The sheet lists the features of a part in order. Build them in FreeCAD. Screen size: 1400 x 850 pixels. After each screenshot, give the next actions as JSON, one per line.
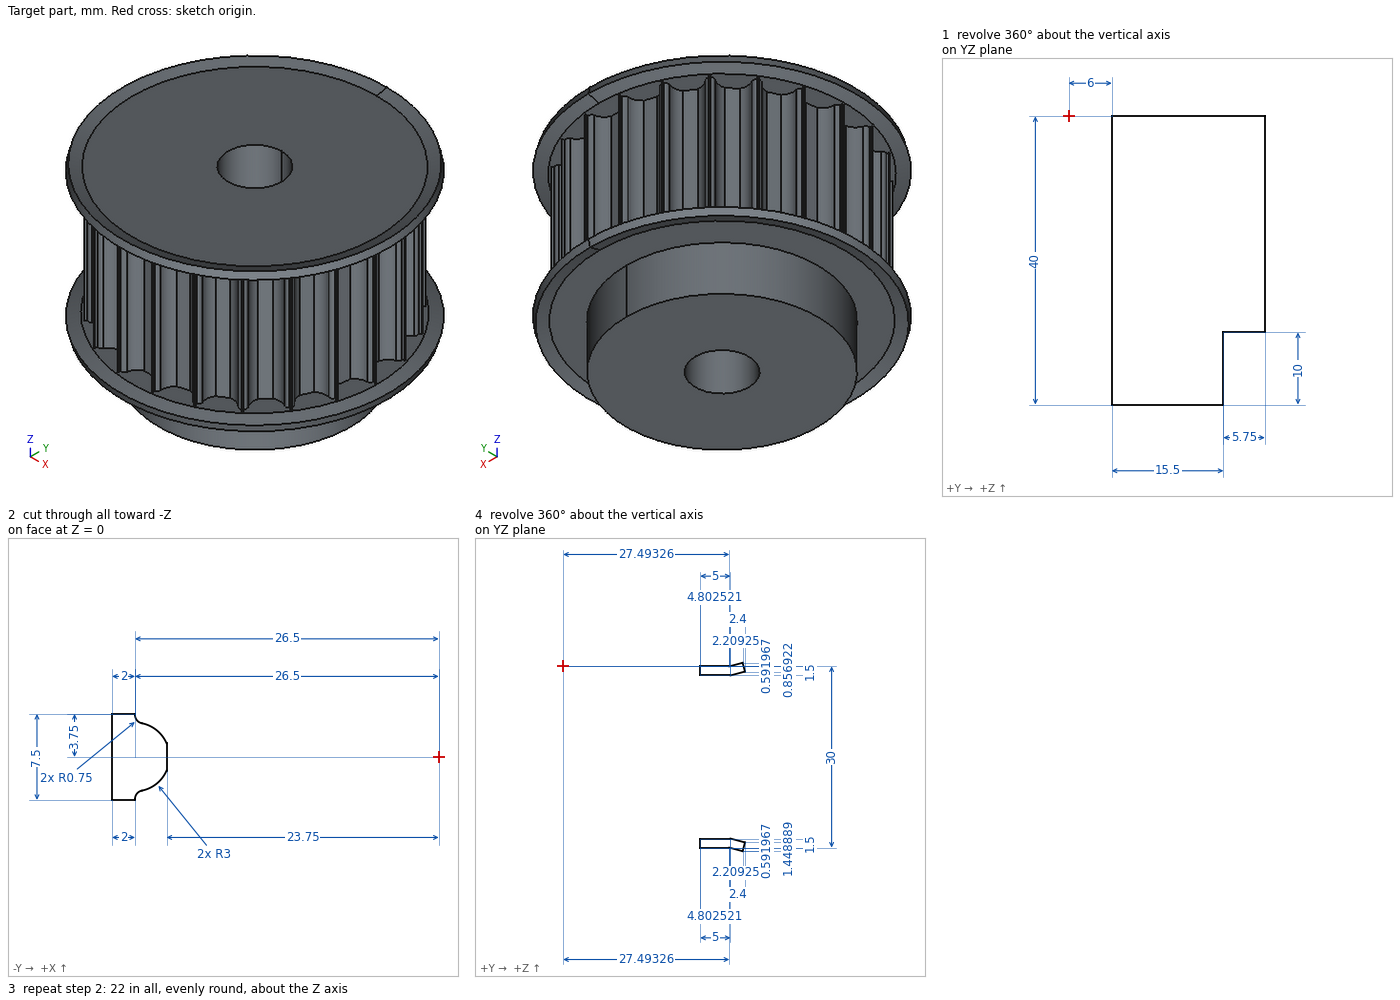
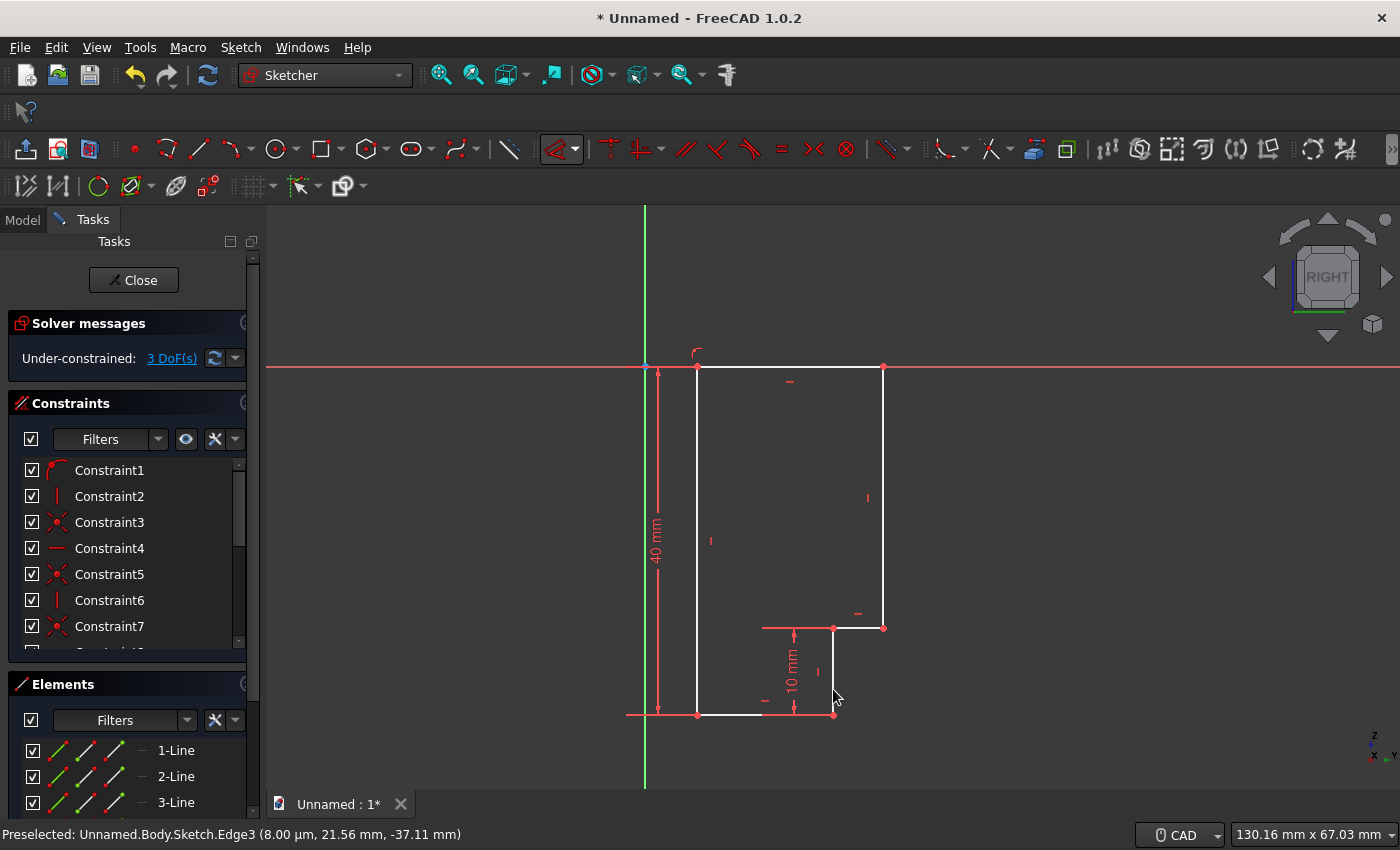
{"action": "left_click", "coordinate": [697, 367]}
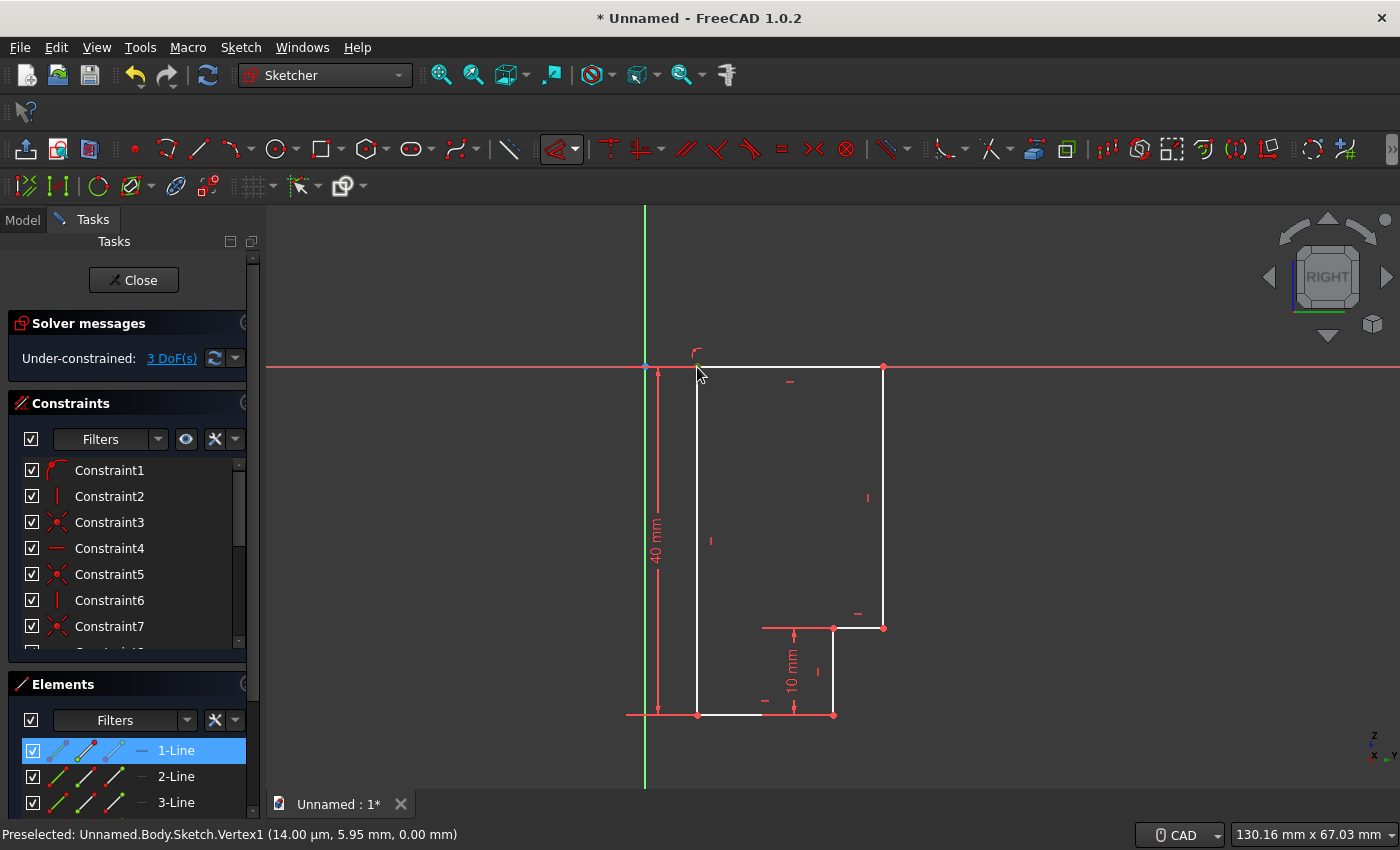
{"action": "left_click", "coordinate": [578, 150]}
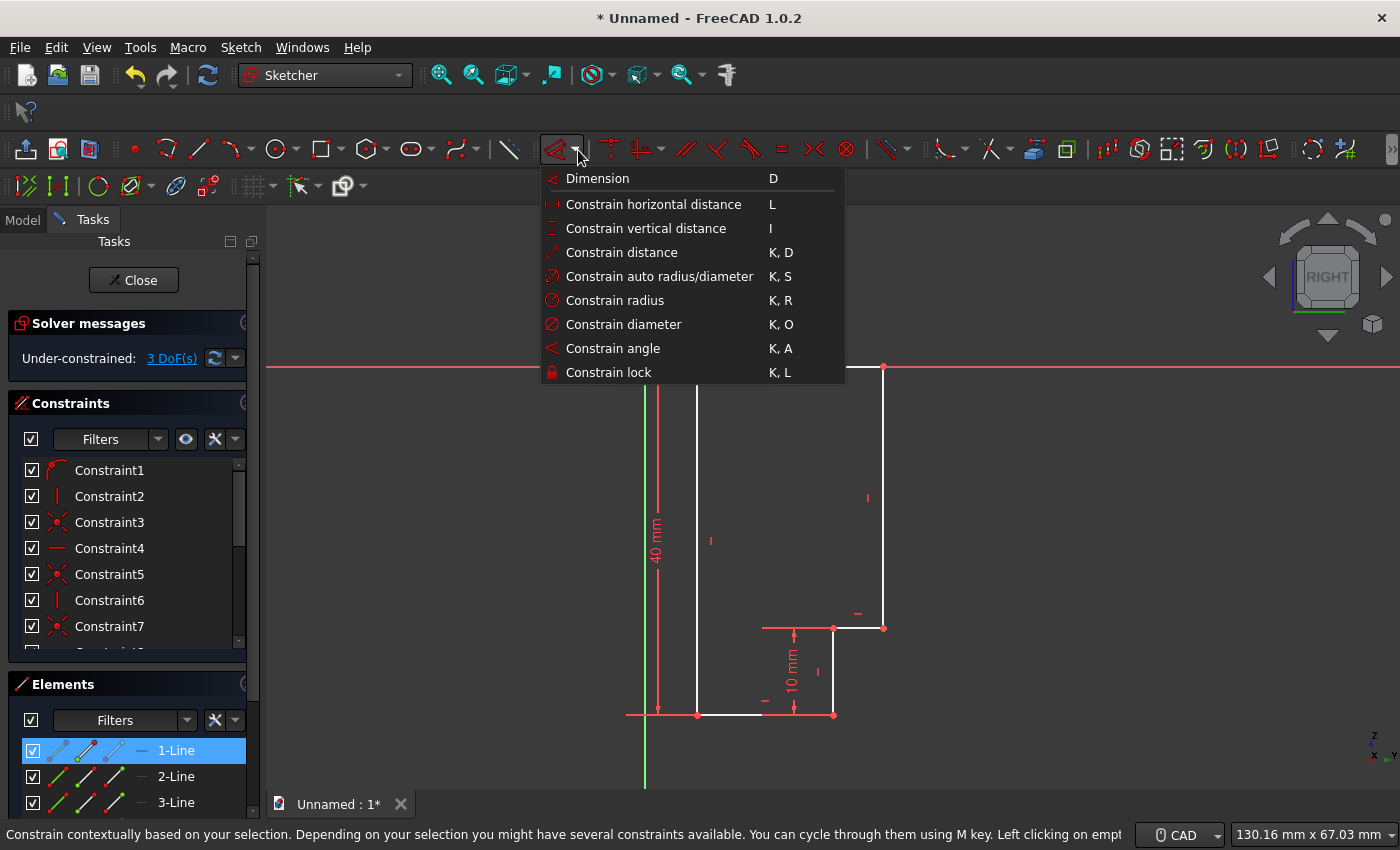
{"action": "left_click", "coordinate": [693, 204]}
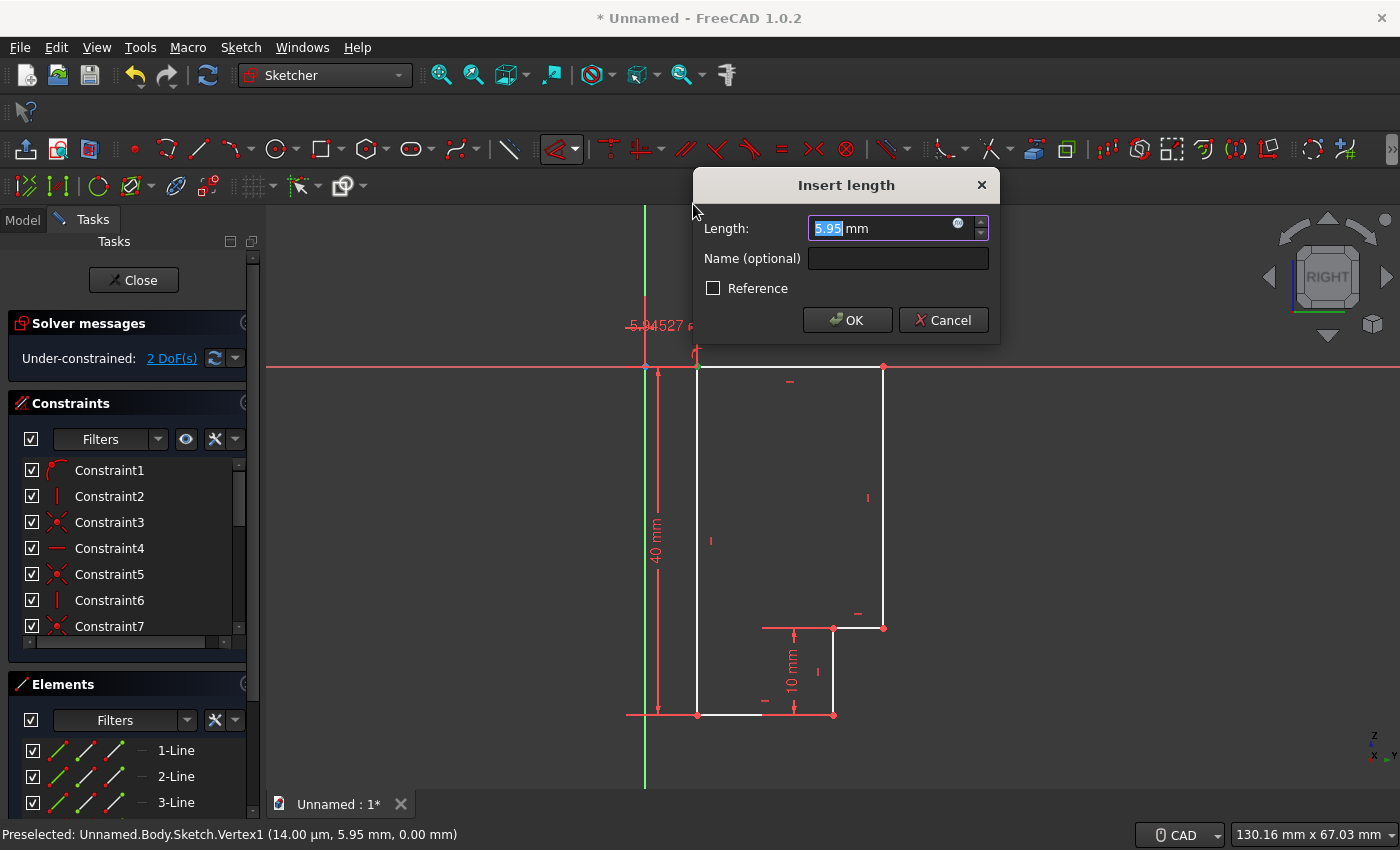
{"action": "type", "text": "6"}
{"action": "key", "text": "Return"}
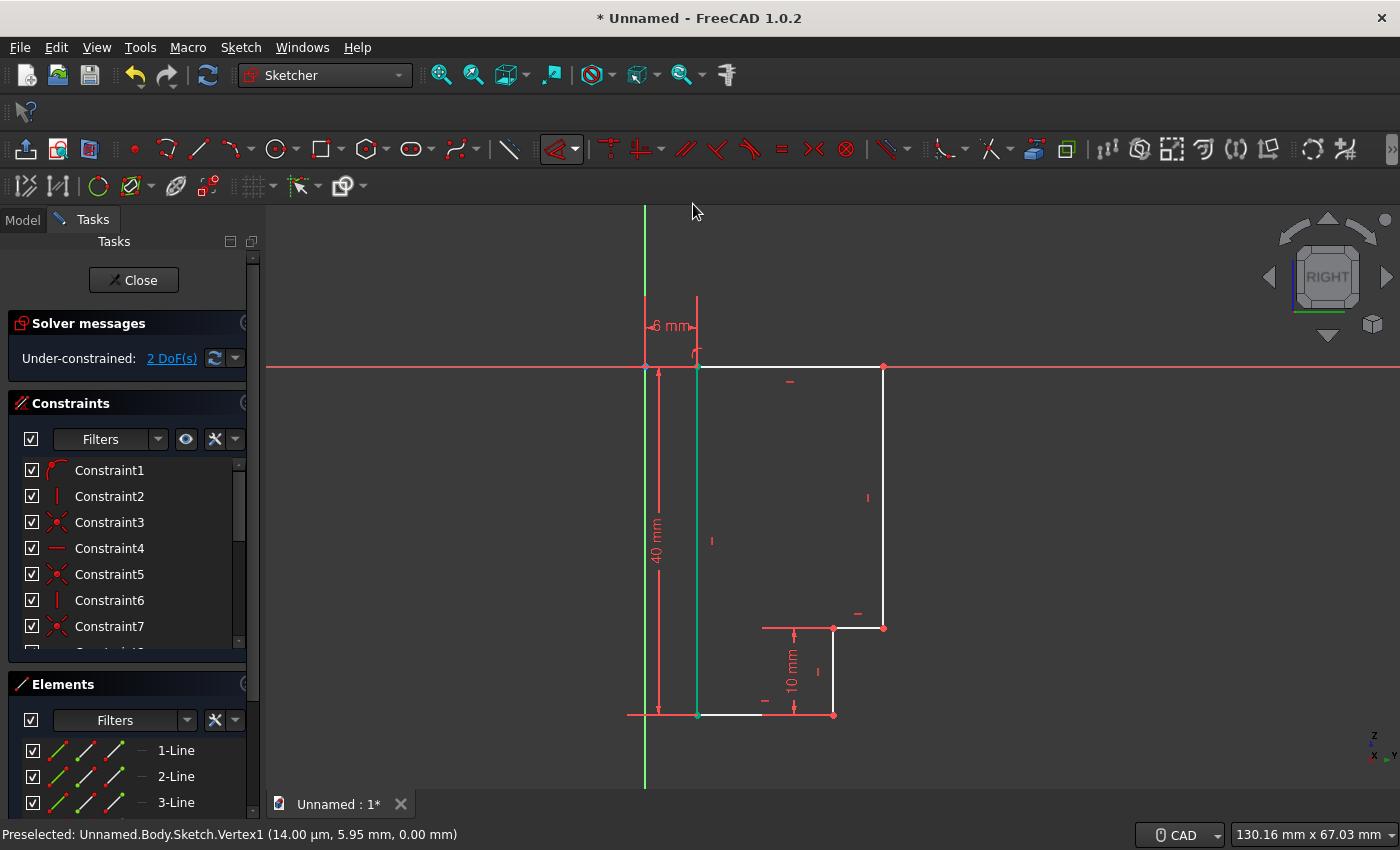
{"action": "left_click", "coordinate": [738, 715]}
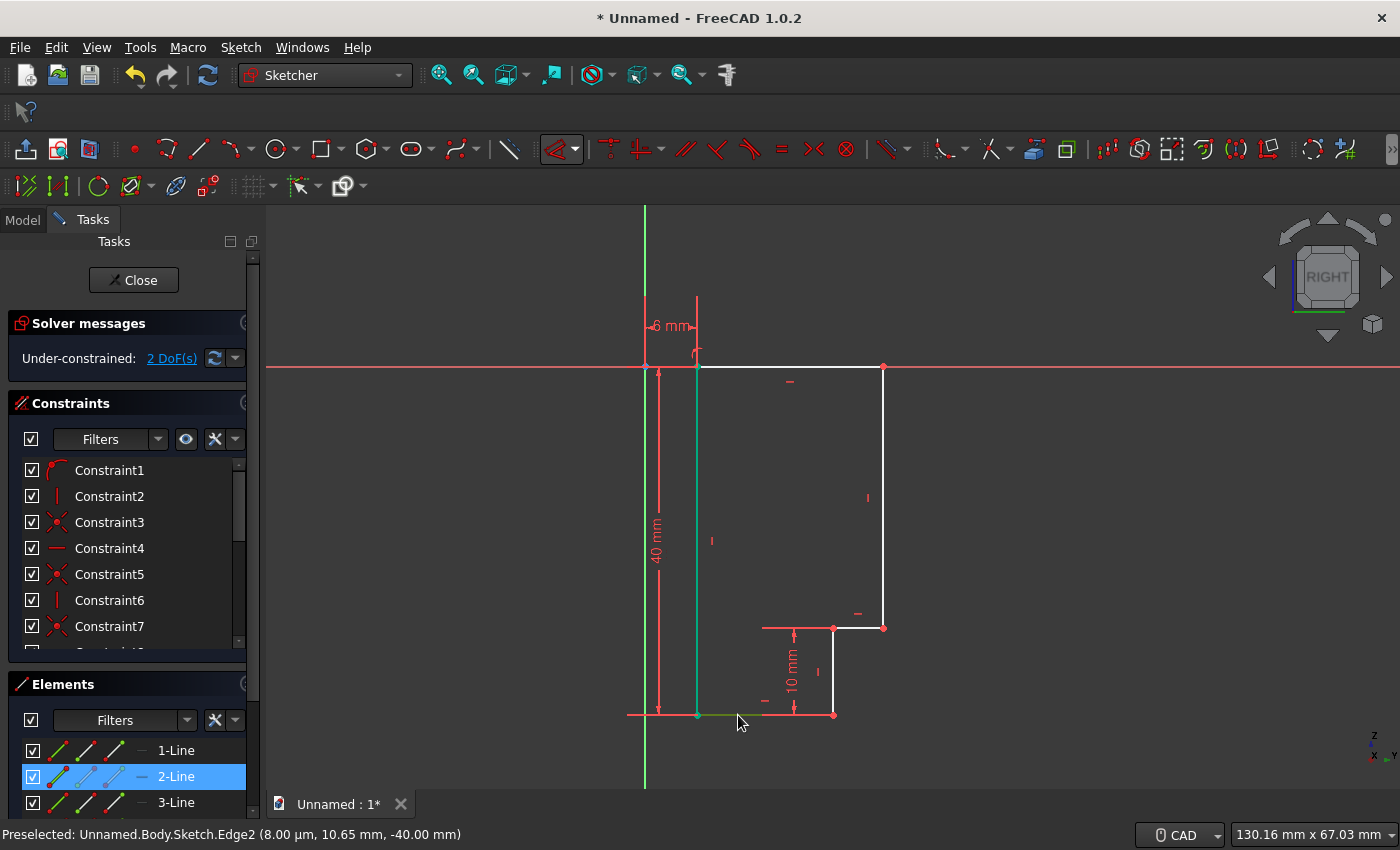
{"action": "left_click", "coordinate": [578, 150]}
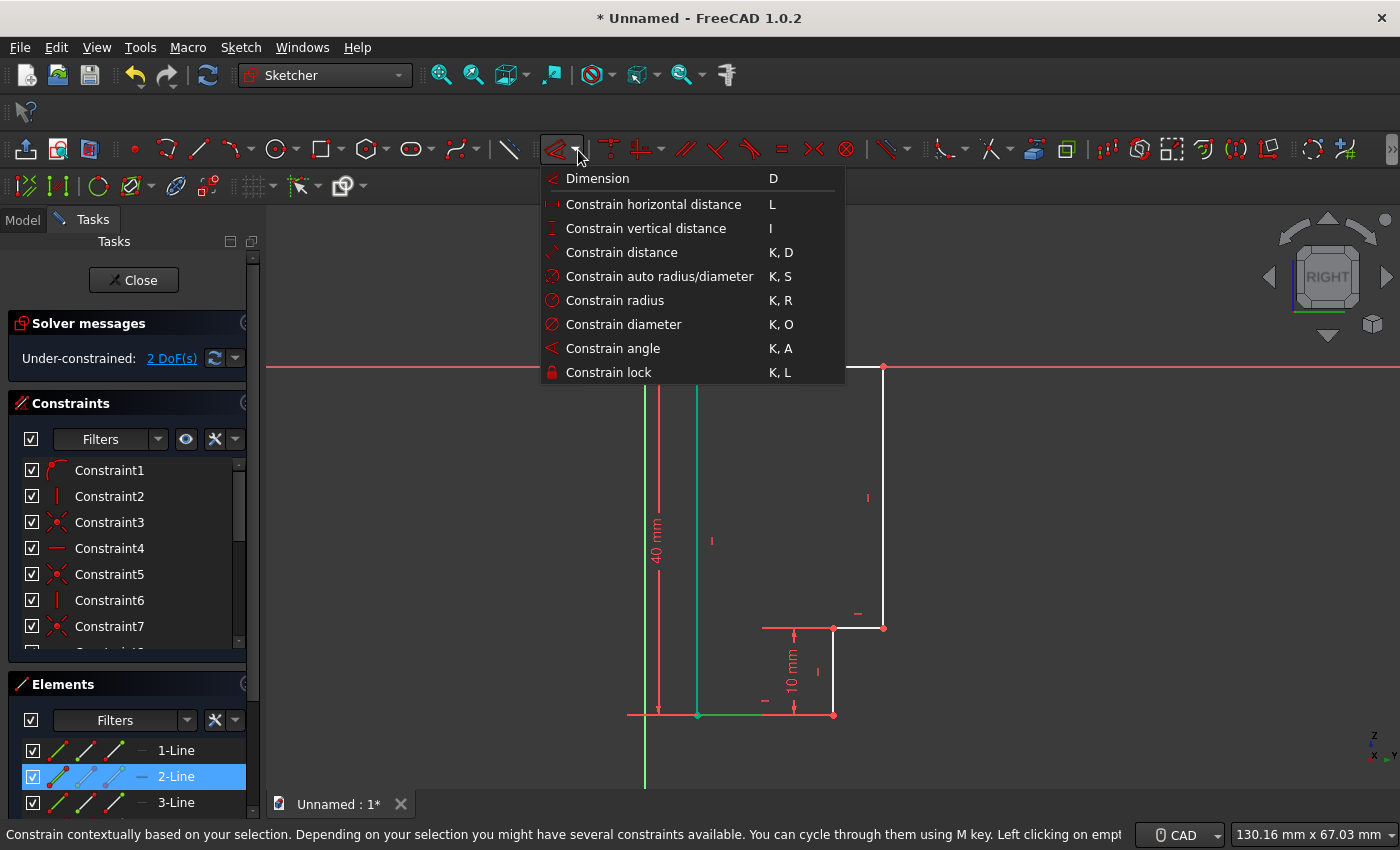
{"action": "left_click", "coordinate": [693, 204]}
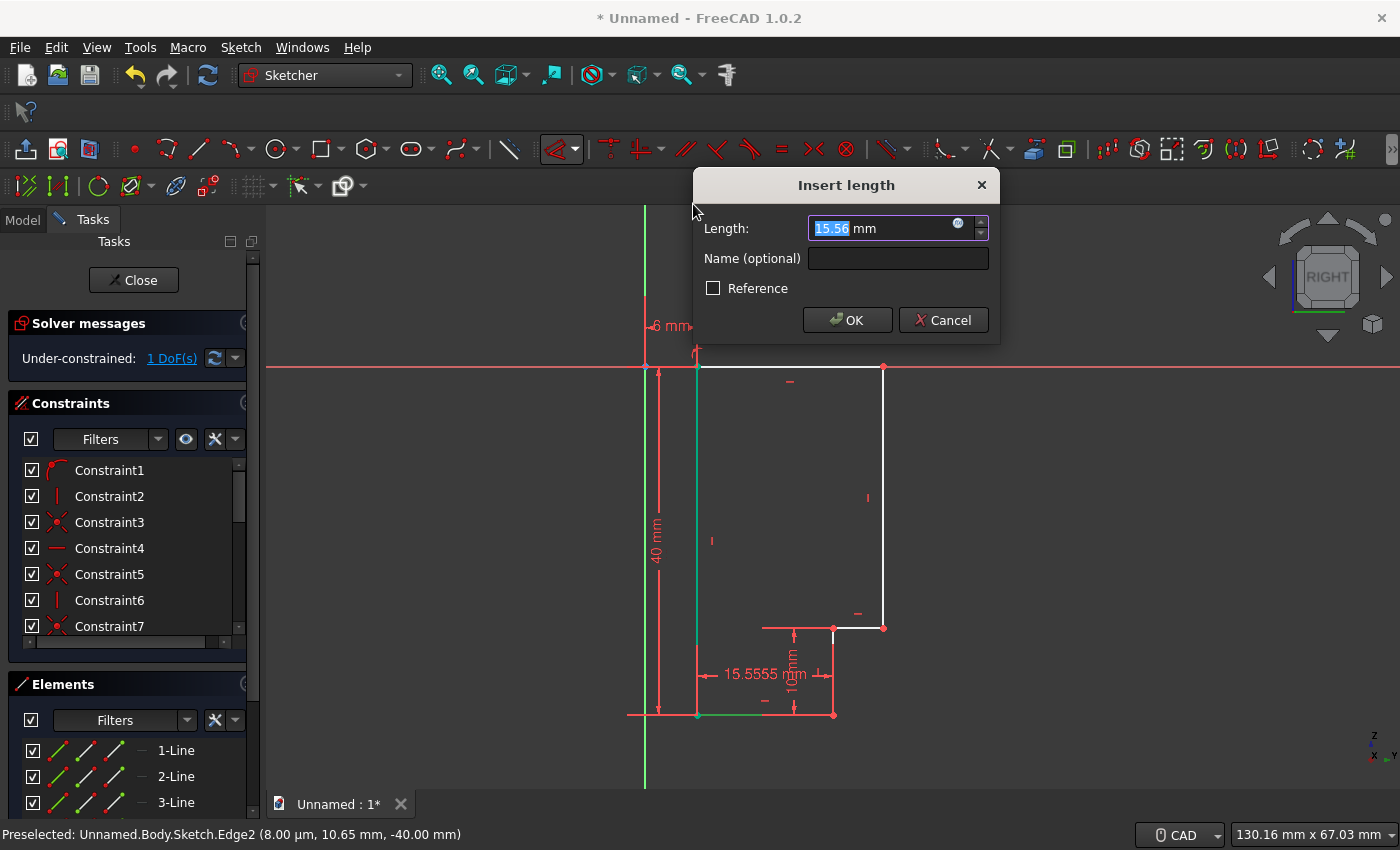
{"action": "type", "text": "15.5"}
{"action": "key", "text": "Return"}